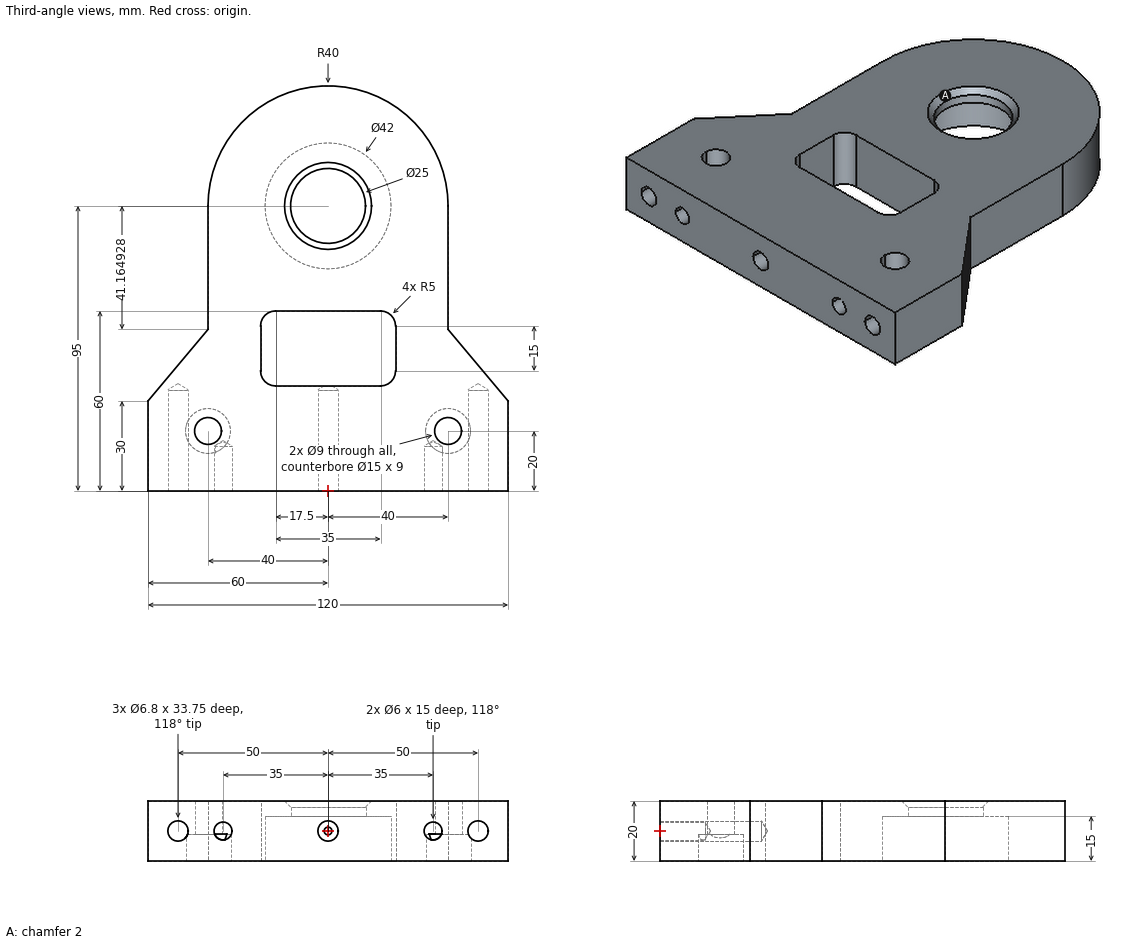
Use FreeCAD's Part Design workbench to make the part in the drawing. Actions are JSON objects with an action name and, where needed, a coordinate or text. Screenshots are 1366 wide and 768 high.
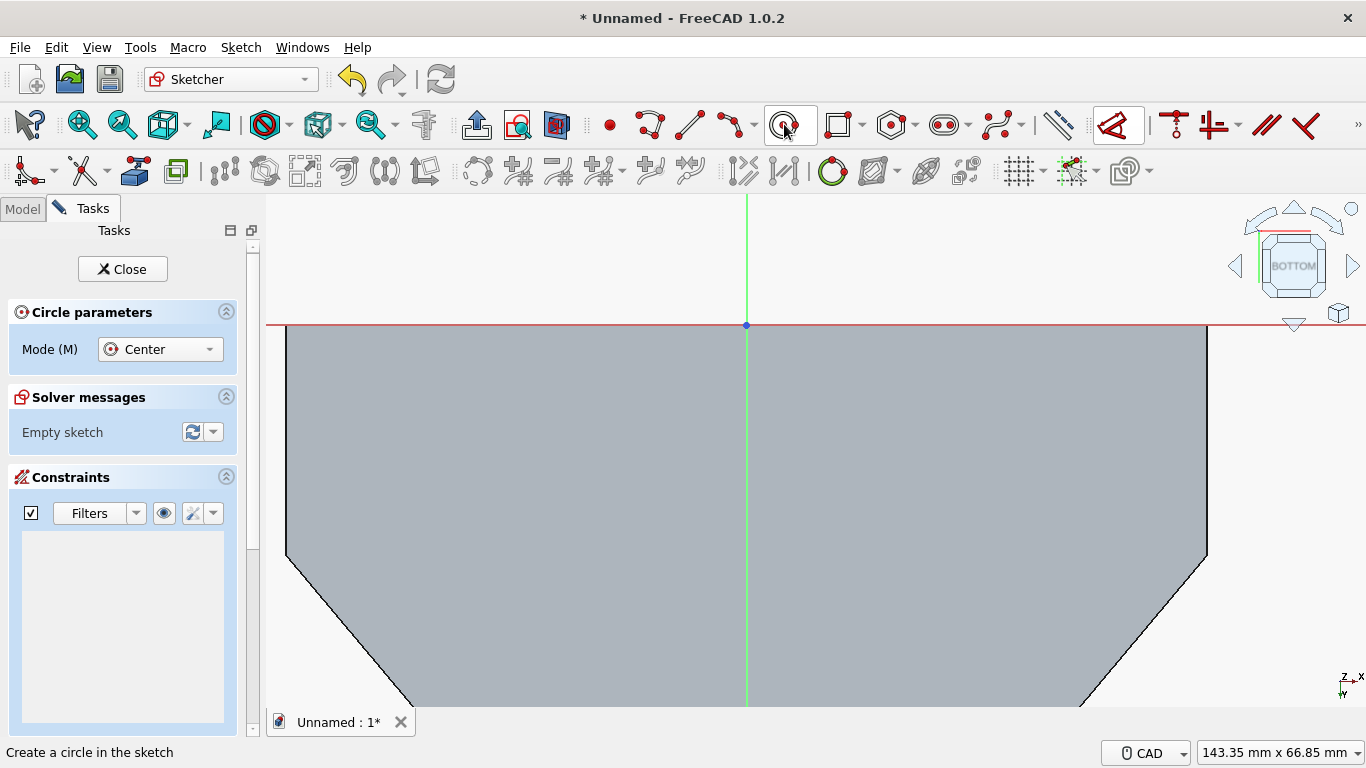
{"action": "left_click", "coordinate": [1054, 479]}
{"action": "left_click", "coordinate": [1078, 454]}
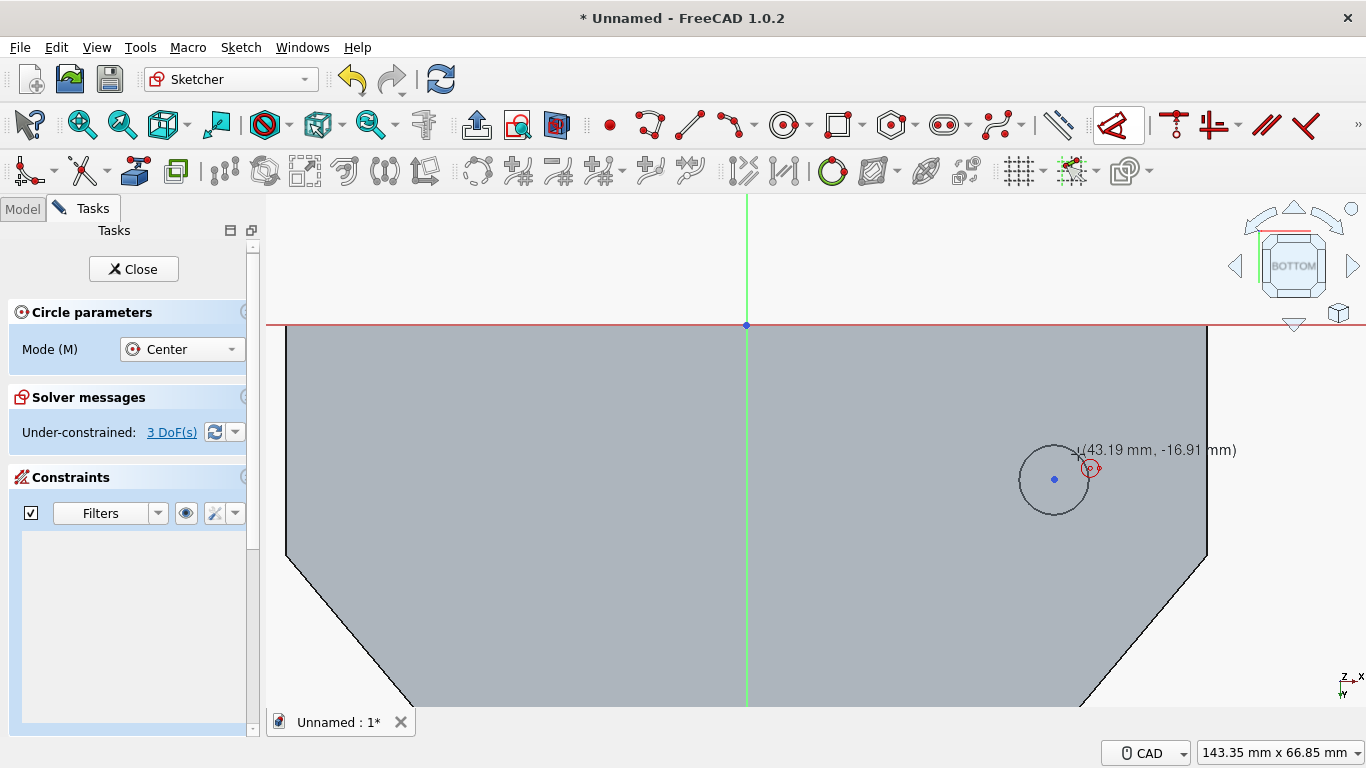
{"action": "left_click", "coordinate": [440, 479]}
{"action": "left_click", "coordinate": [464, 454]}
{"action": "key", "text": "Escape"}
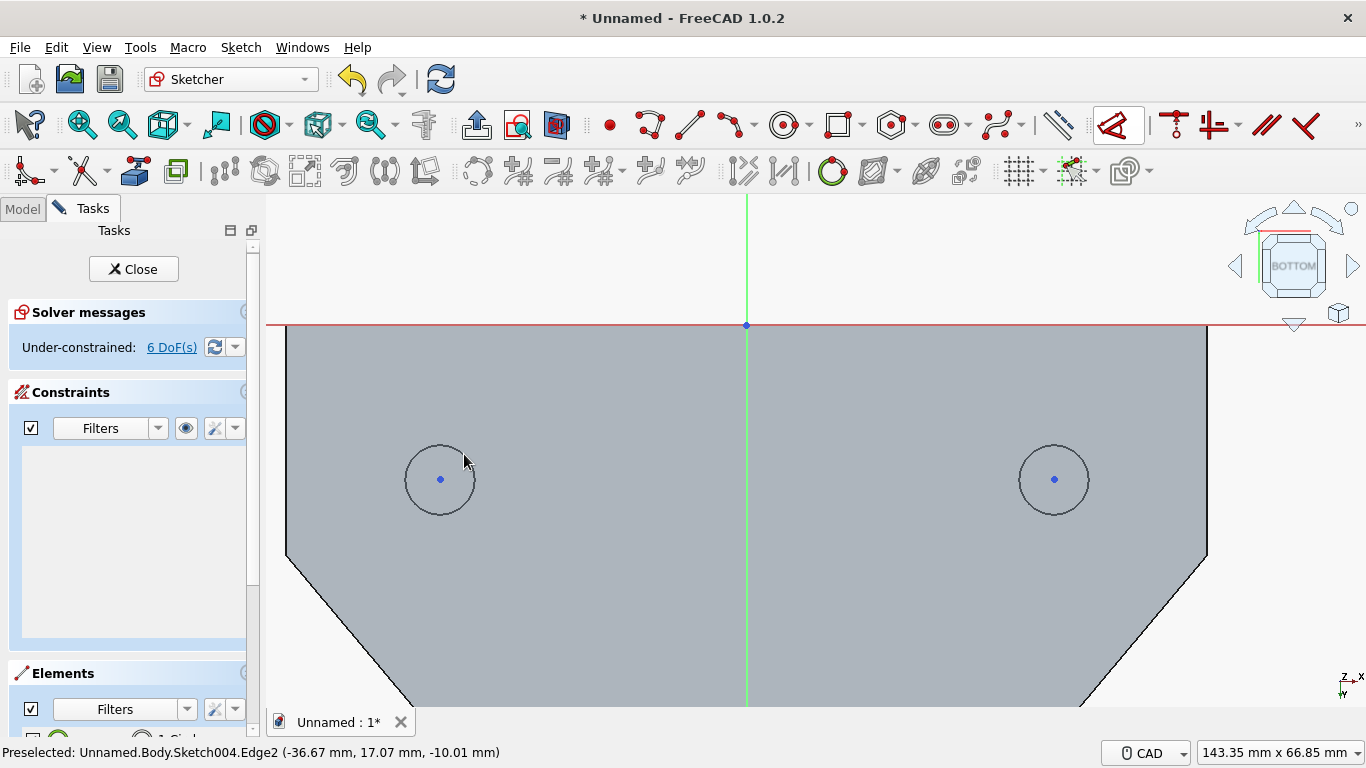
{"action": "left_click", "coordinate": [1078, 455]}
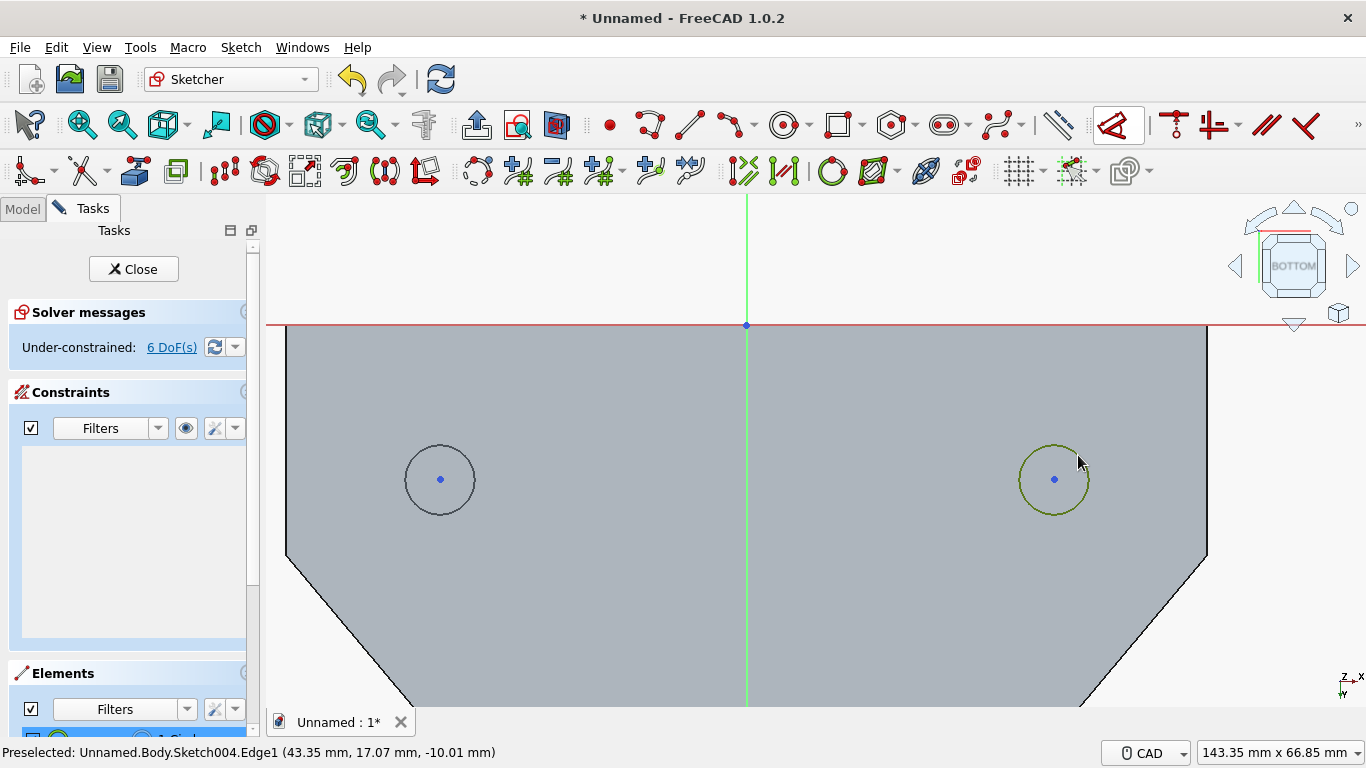
{"action": "left_click", "coordinate": [464, 455]}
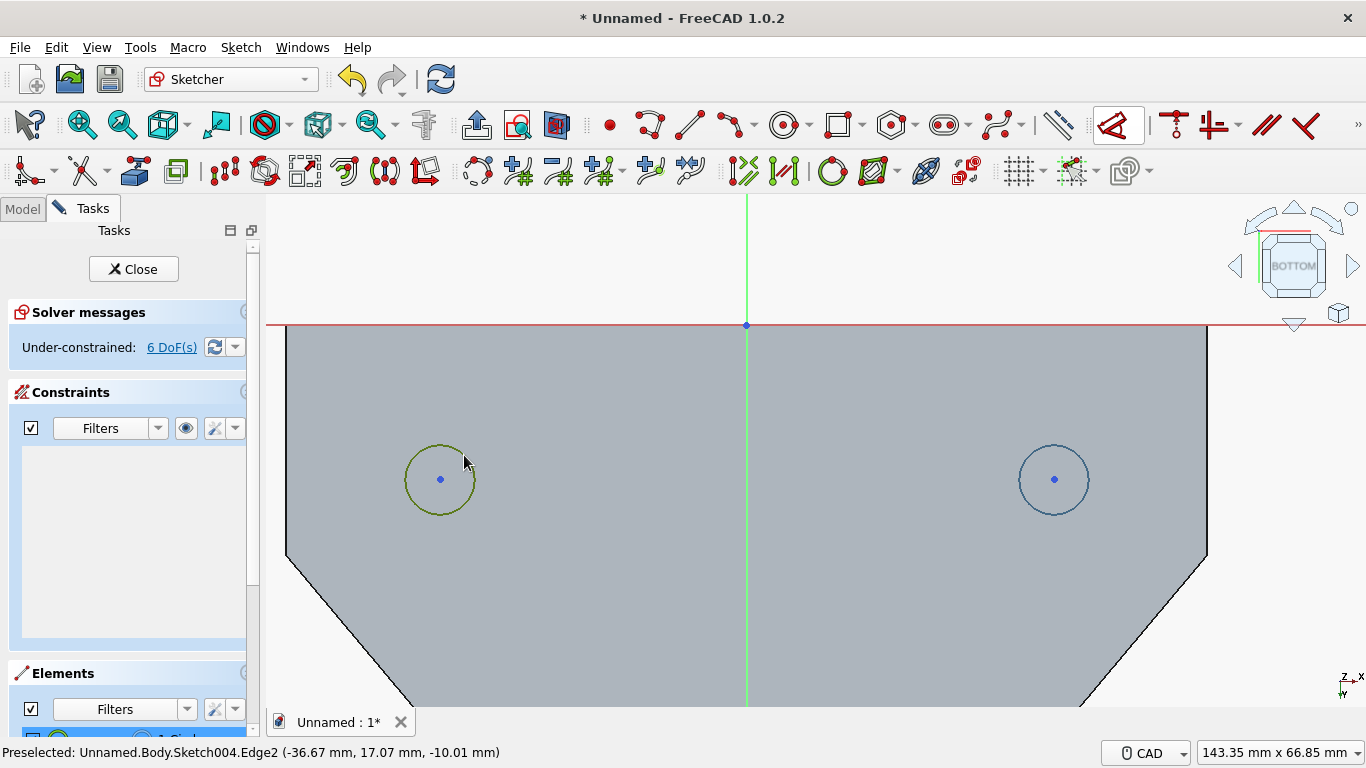
{"action": "key", "text": "e"}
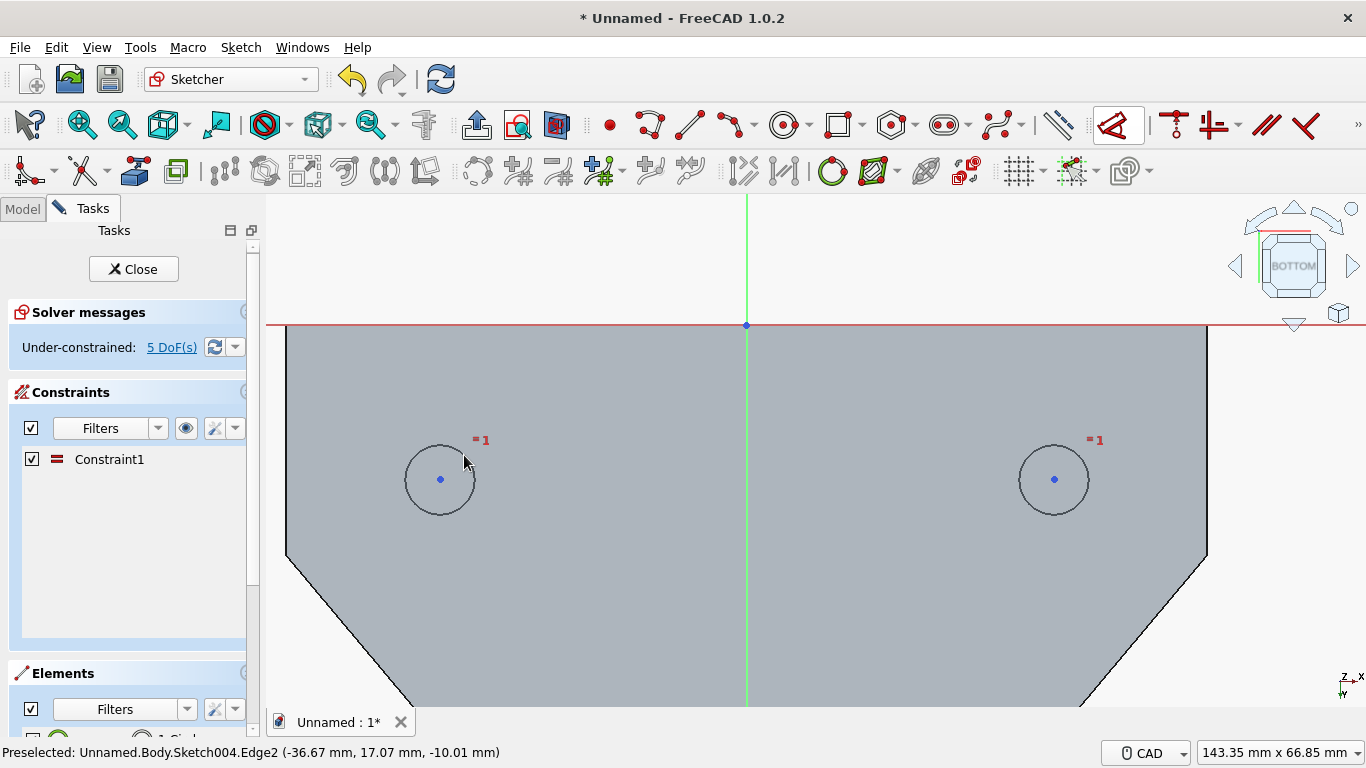
{"action": "left_click", "coordinate": [1078, 455]}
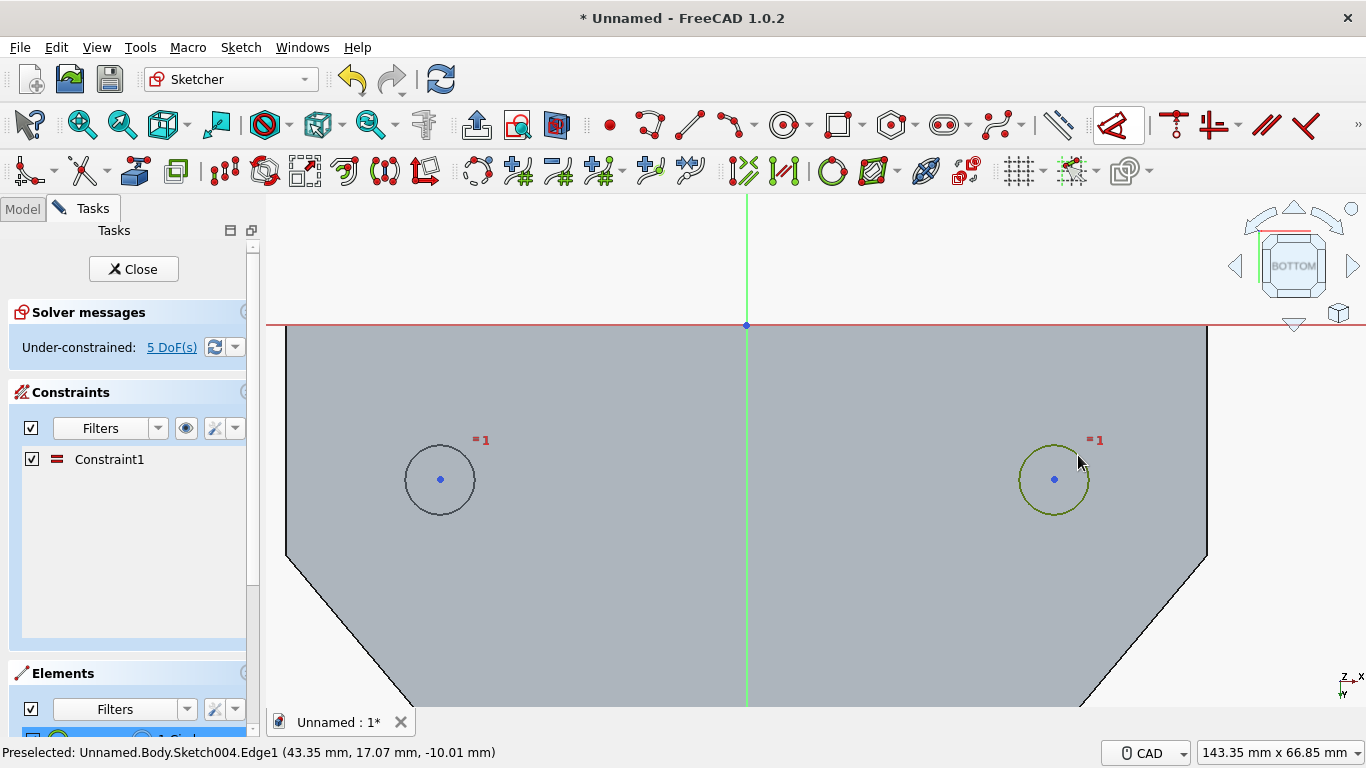
{"action": "key", "text": "k o"}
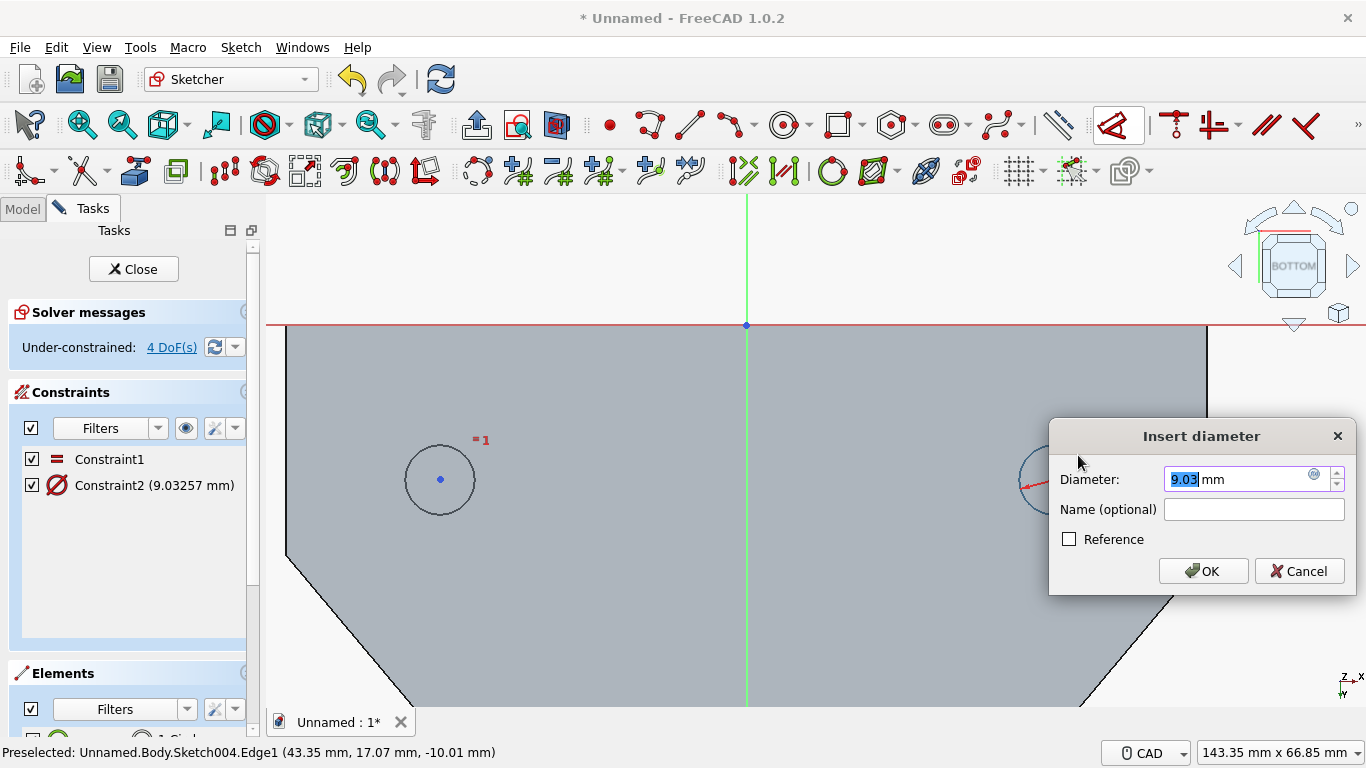
{"action": "type", "text": "9"}
{"action": "key", "text": "Return"}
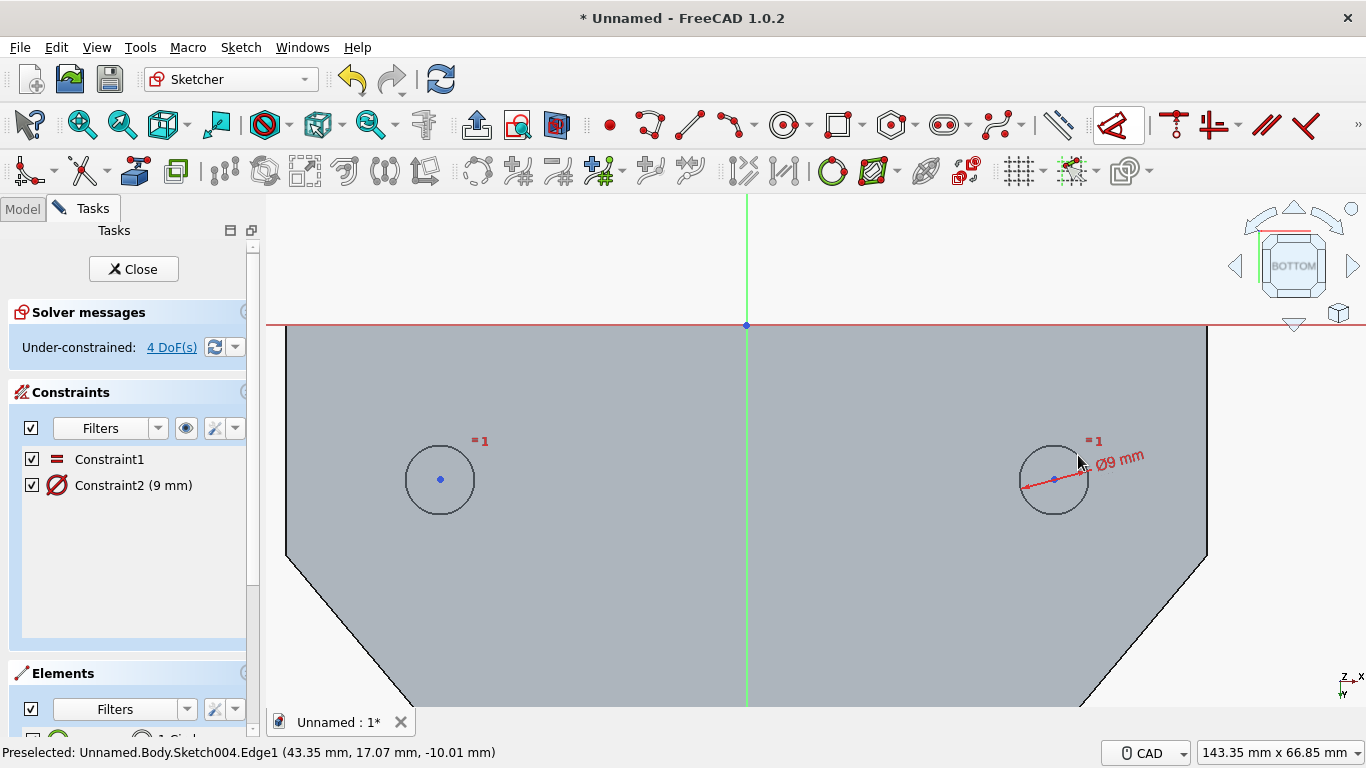
{"action": "left_click", "coordinate": [1054, 480]}